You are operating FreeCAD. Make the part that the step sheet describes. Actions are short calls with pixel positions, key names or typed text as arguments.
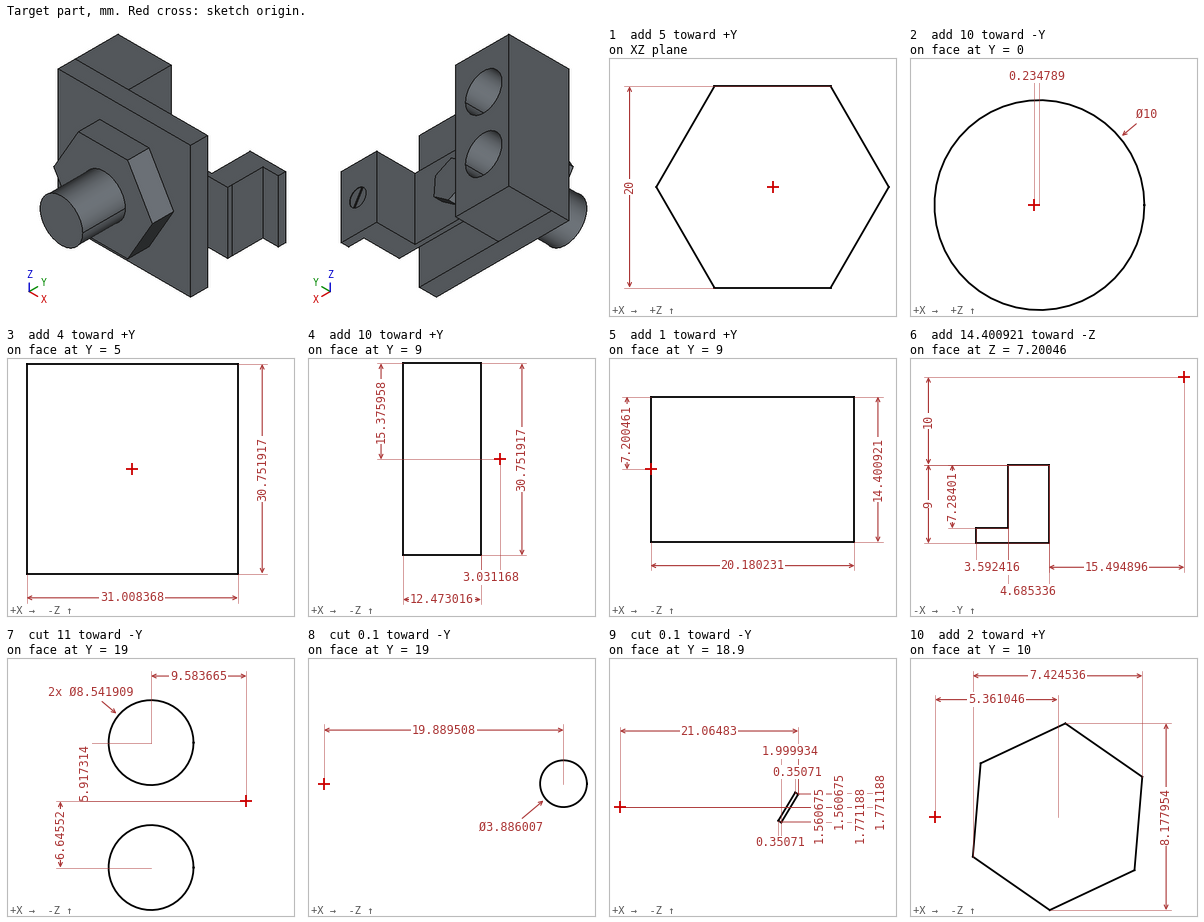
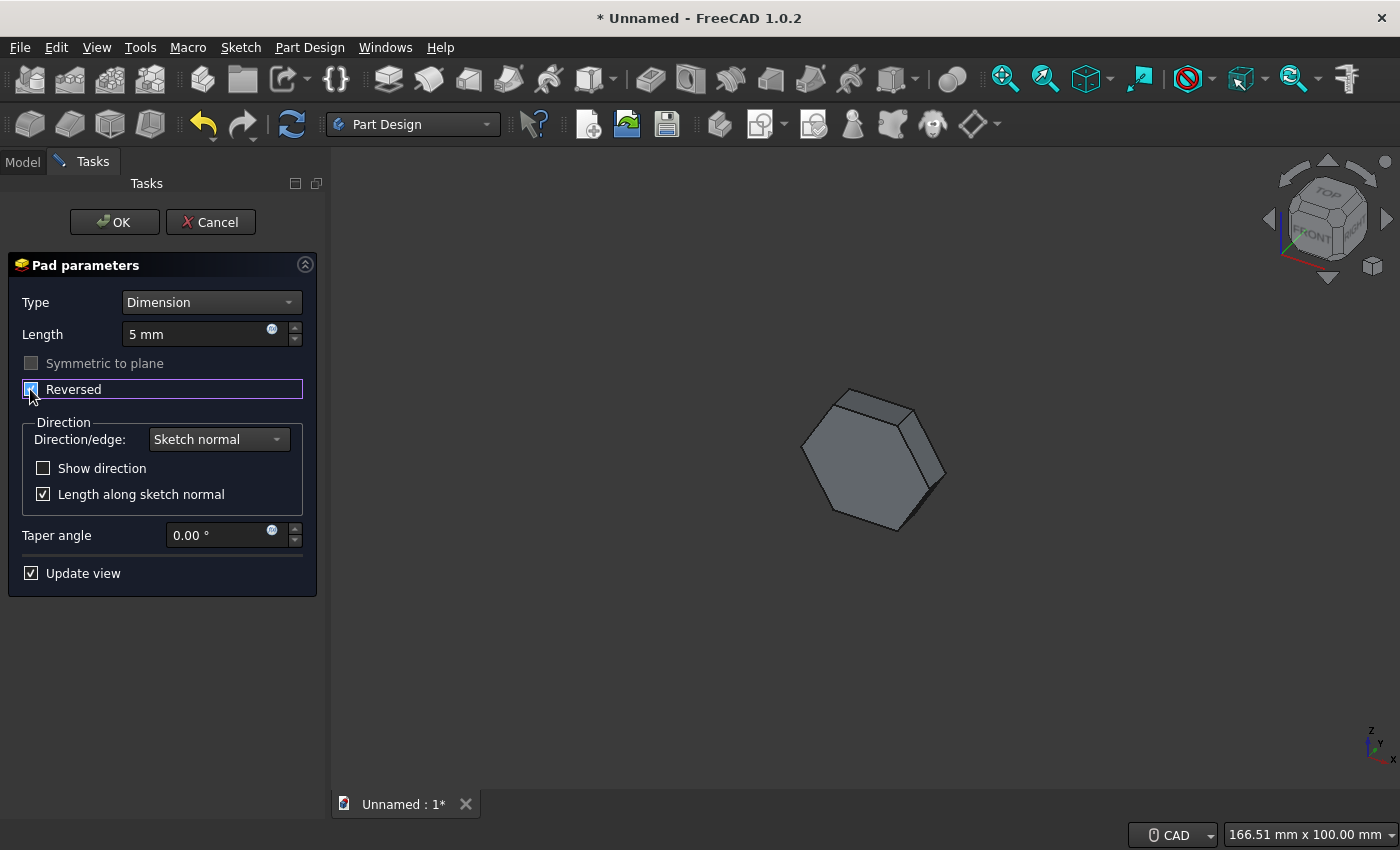
click(115, 222)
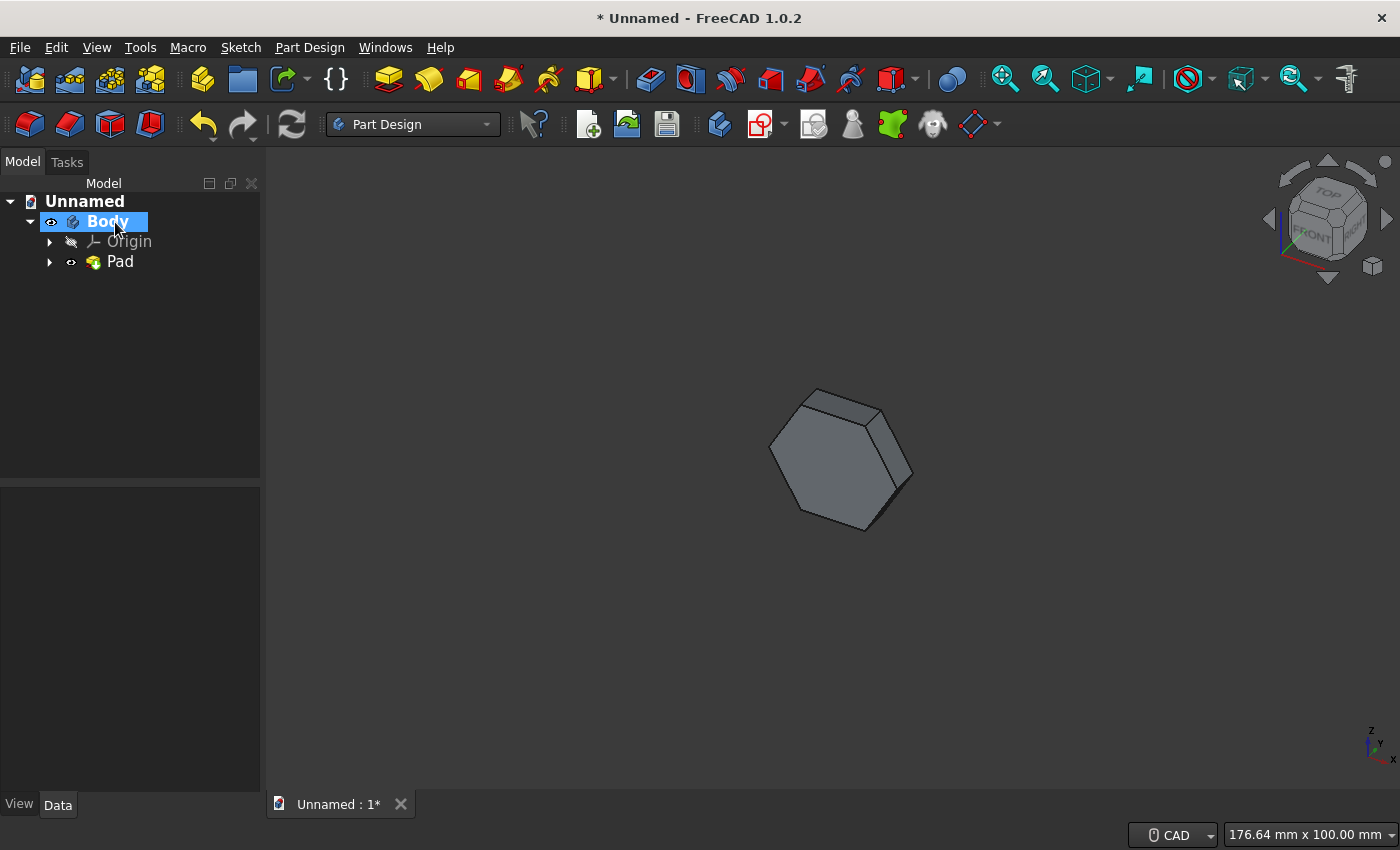
click(1006, 80)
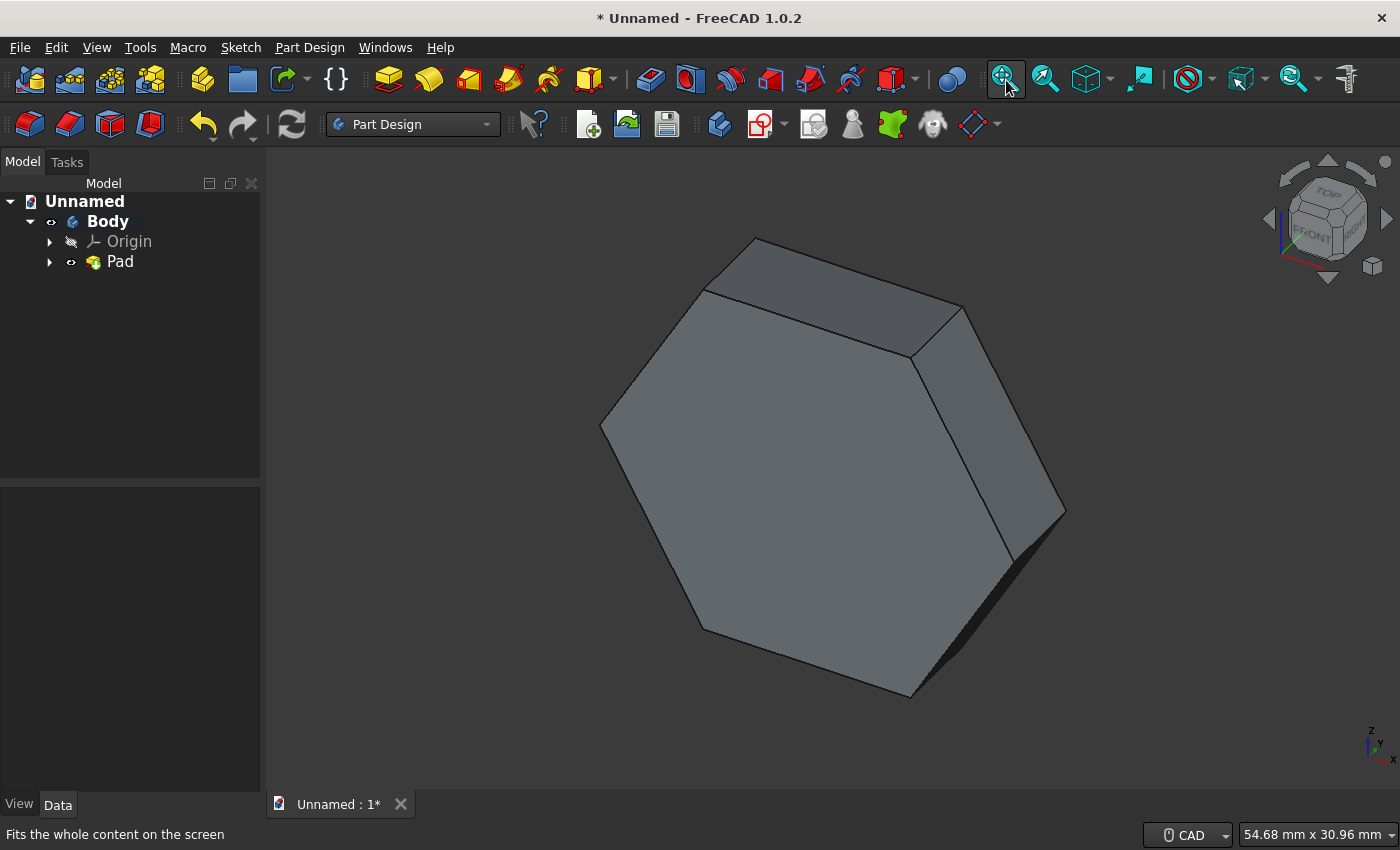
click(807, 493)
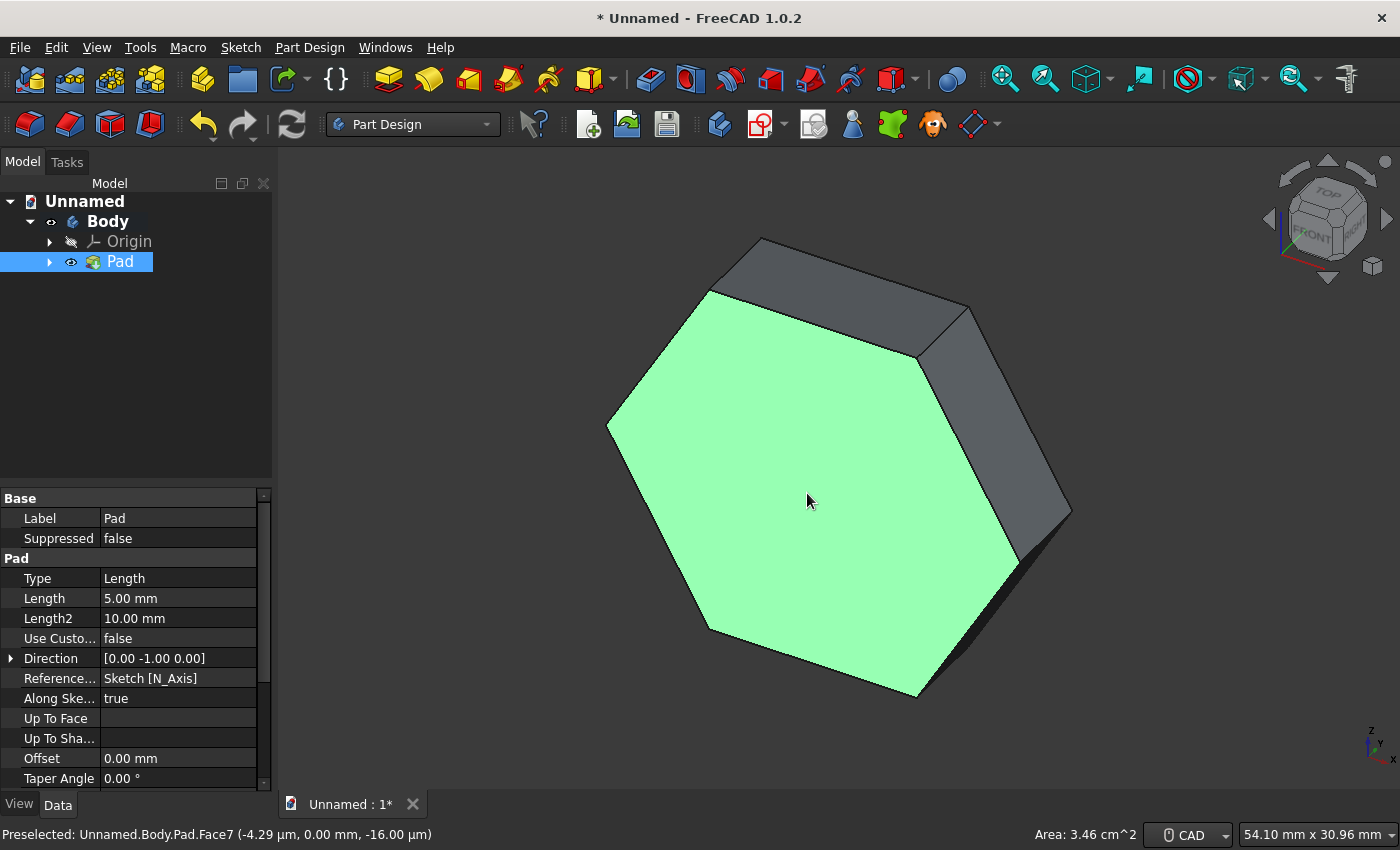
click(760, 124)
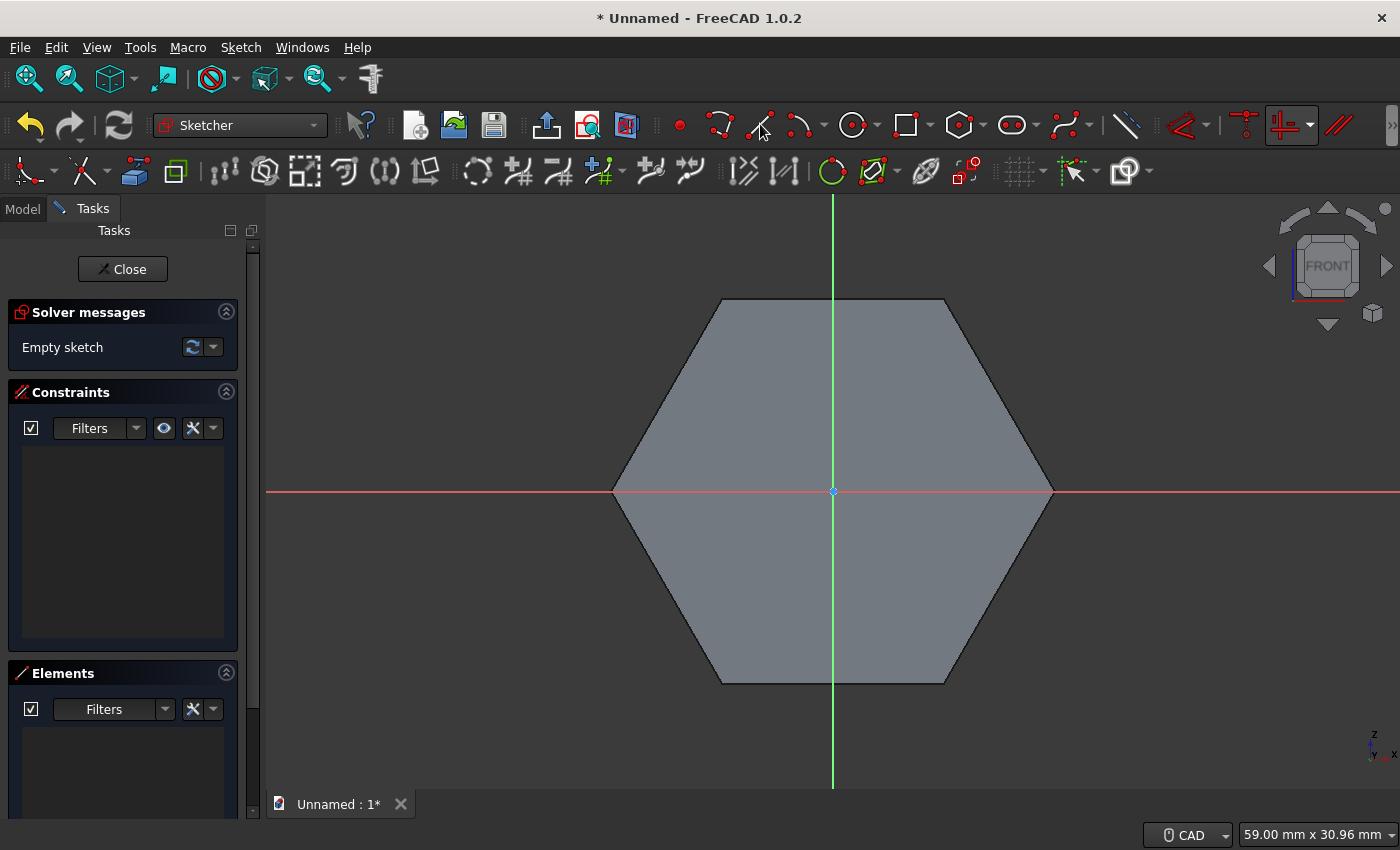
scroll(926, 492, up, 3)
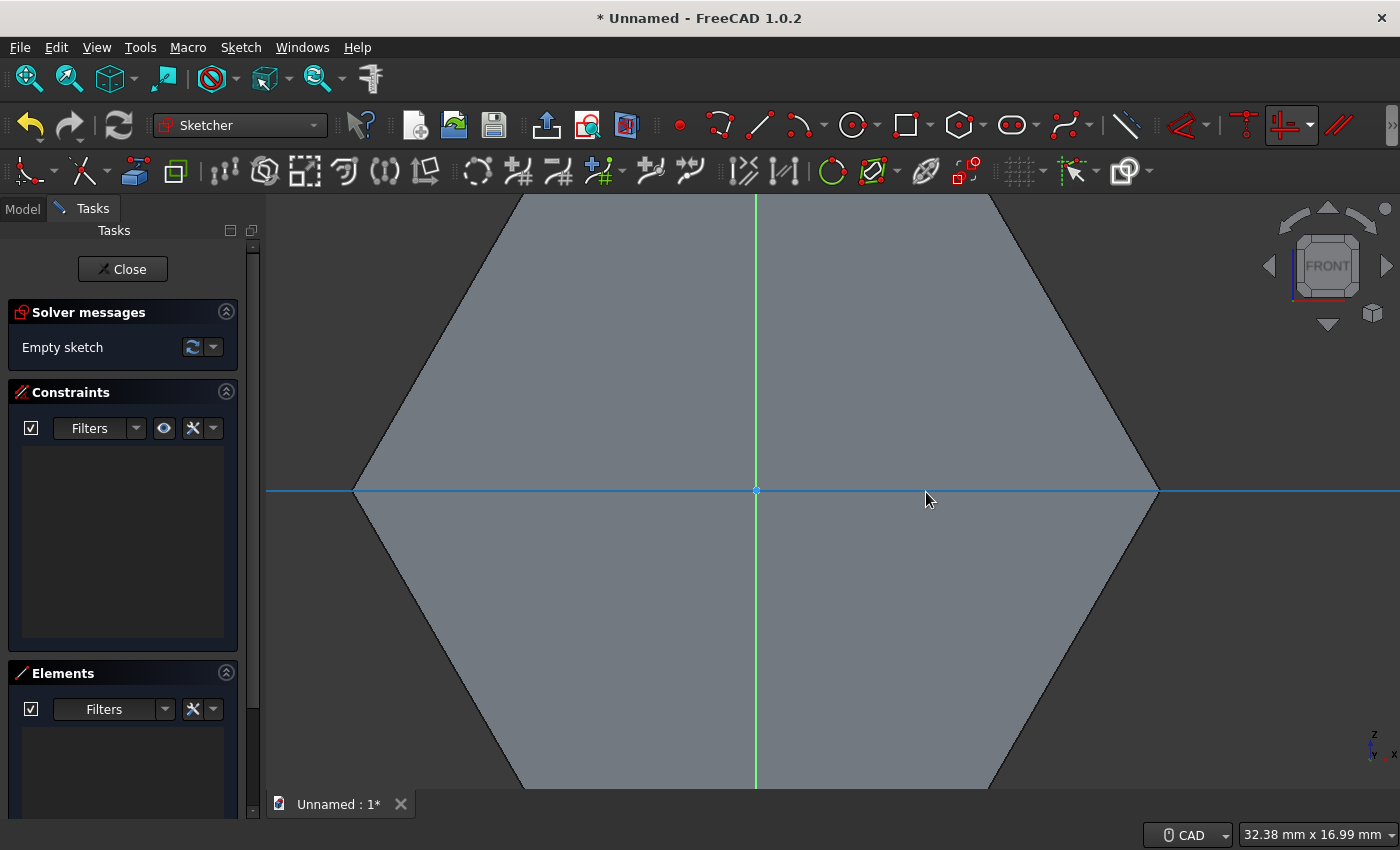
click(854, 126)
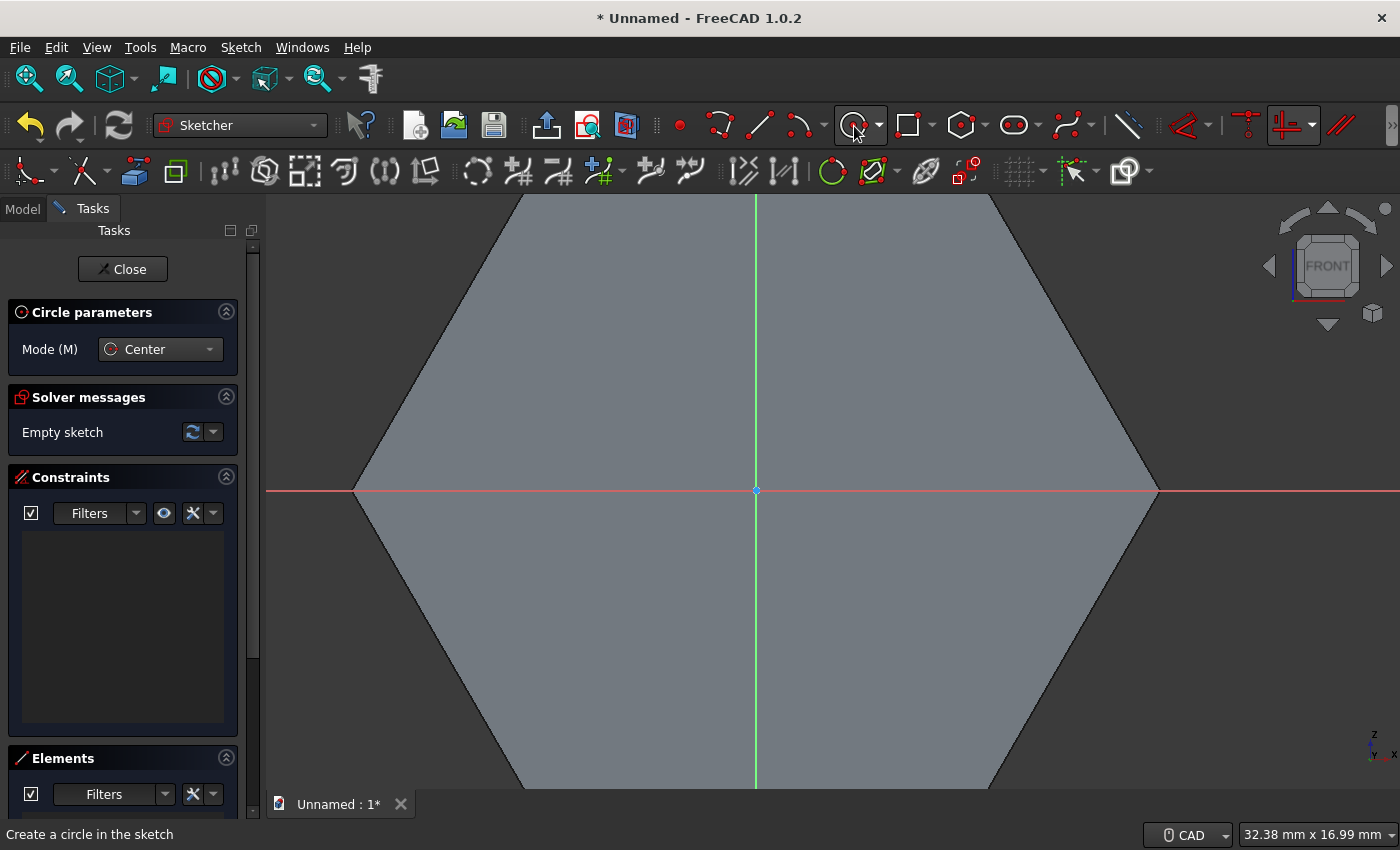
scroll(764, 491, up, 4)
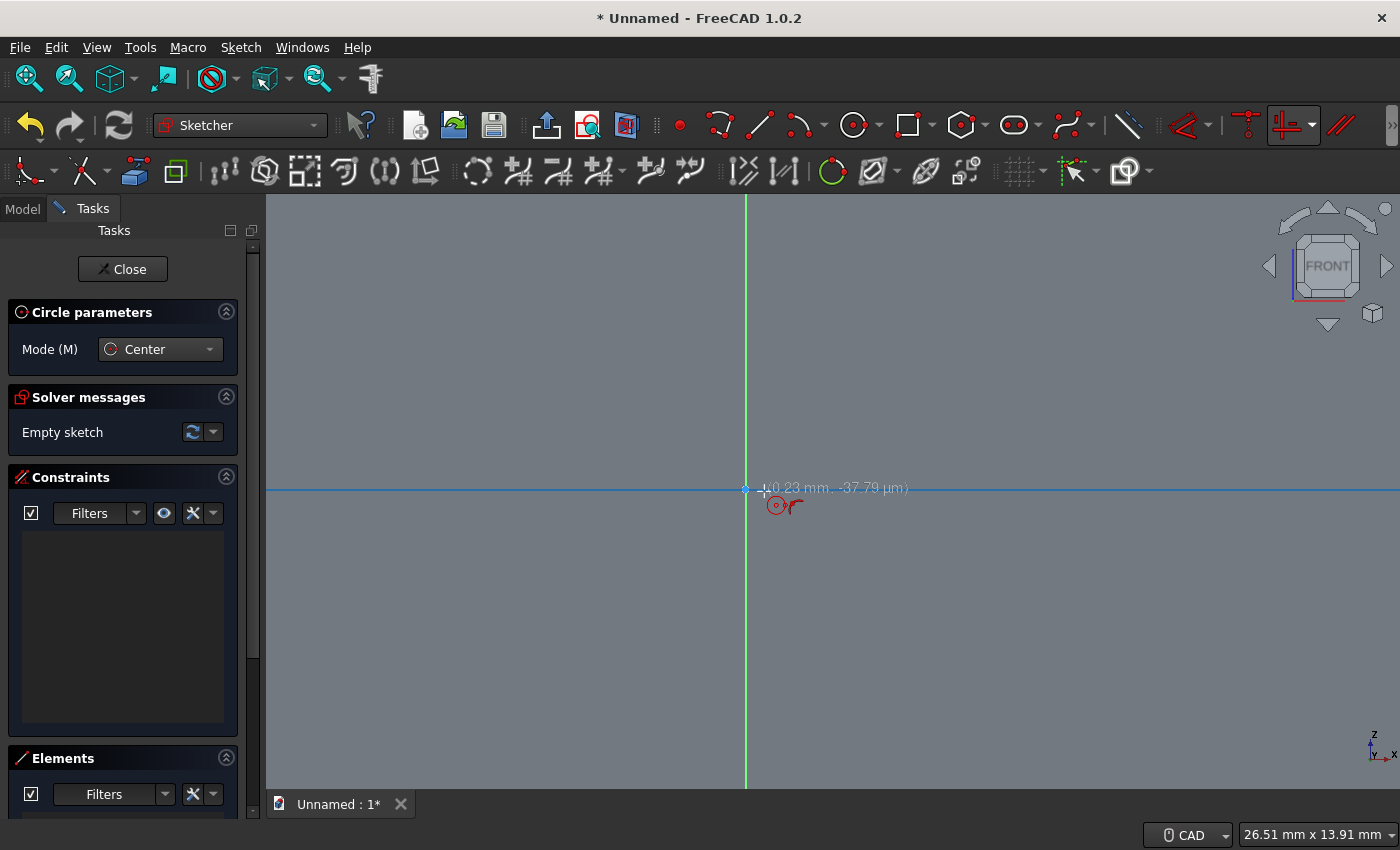
click(764, 490)